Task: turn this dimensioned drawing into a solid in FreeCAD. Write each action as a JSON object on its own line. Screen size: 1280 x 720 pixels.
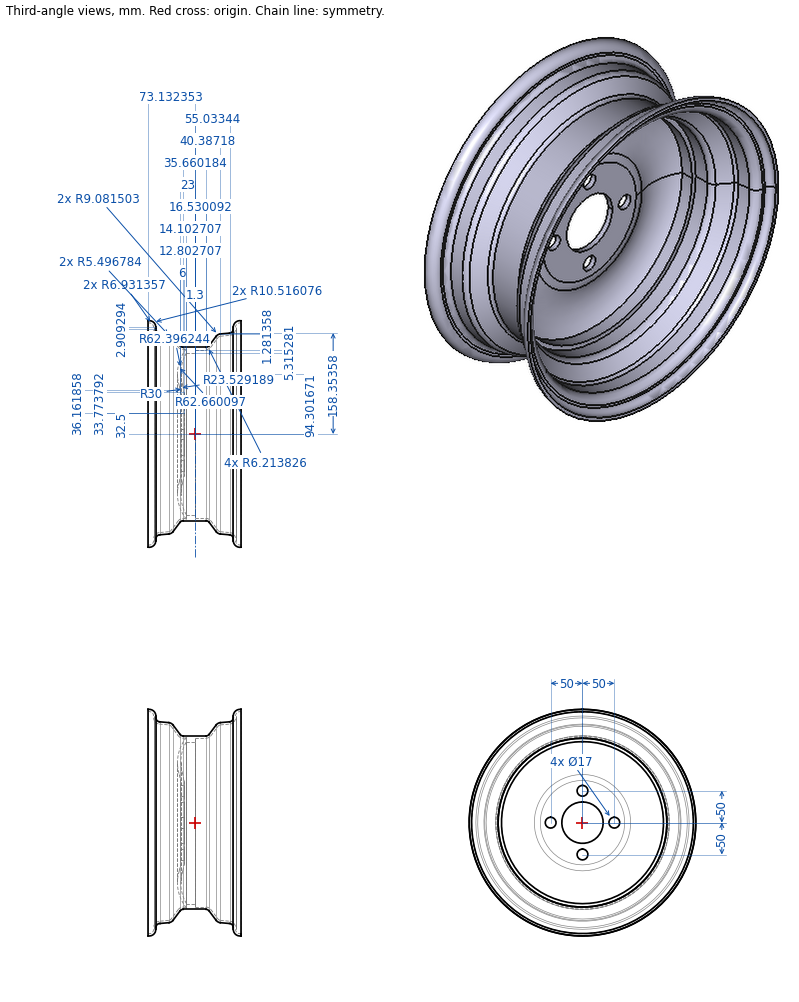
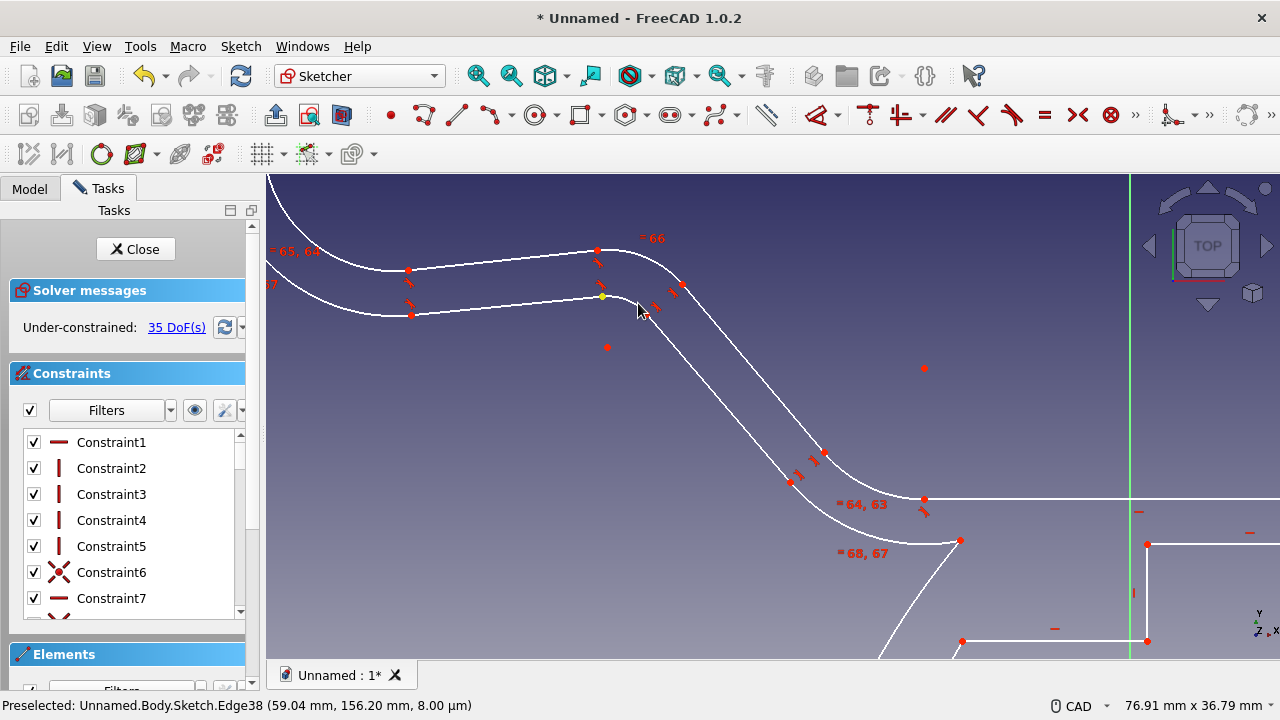
{"action": "left_click", "coordinate": [636, 305]}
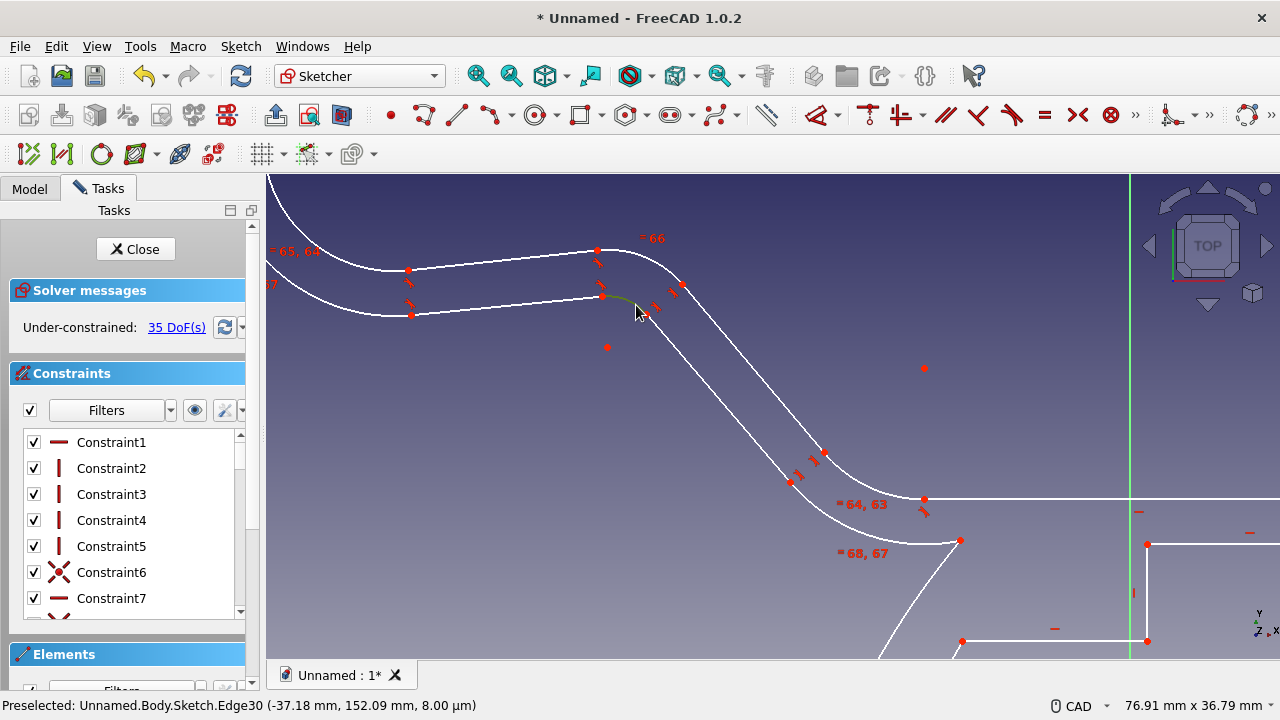
{"action": "scroll", "coordinate": [638, 303], "scroll_direction": "down", "scroll_amount": 10}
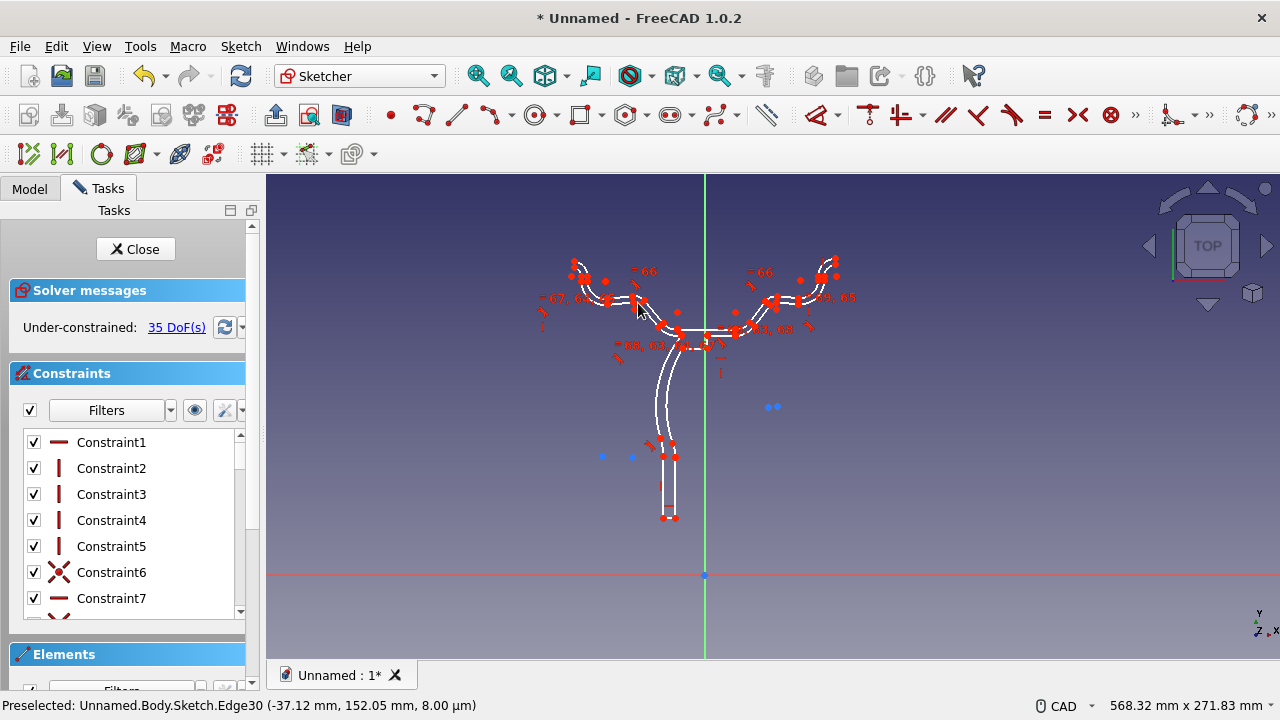
{"action": "scroll", "coordinate": [775, 303], "scroll_direction": "up", "scroll_amount": 10}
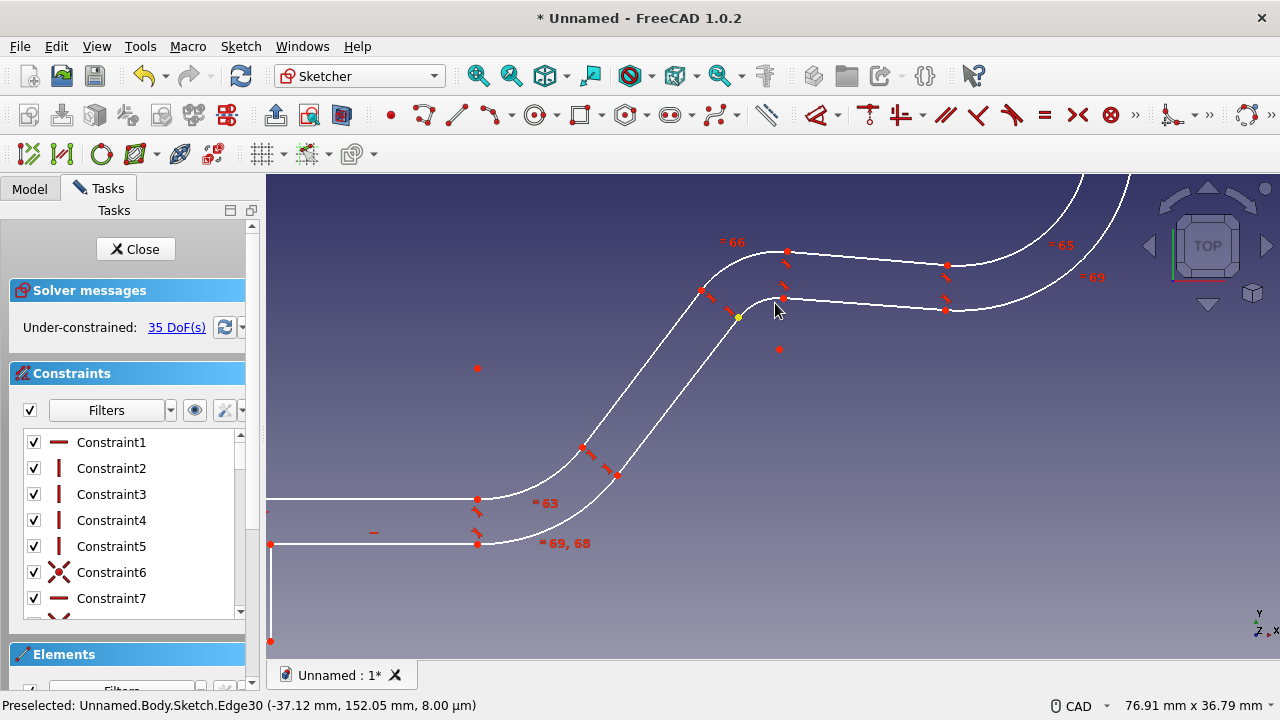
{"action": "left_click", "coordinate": [768, 299]}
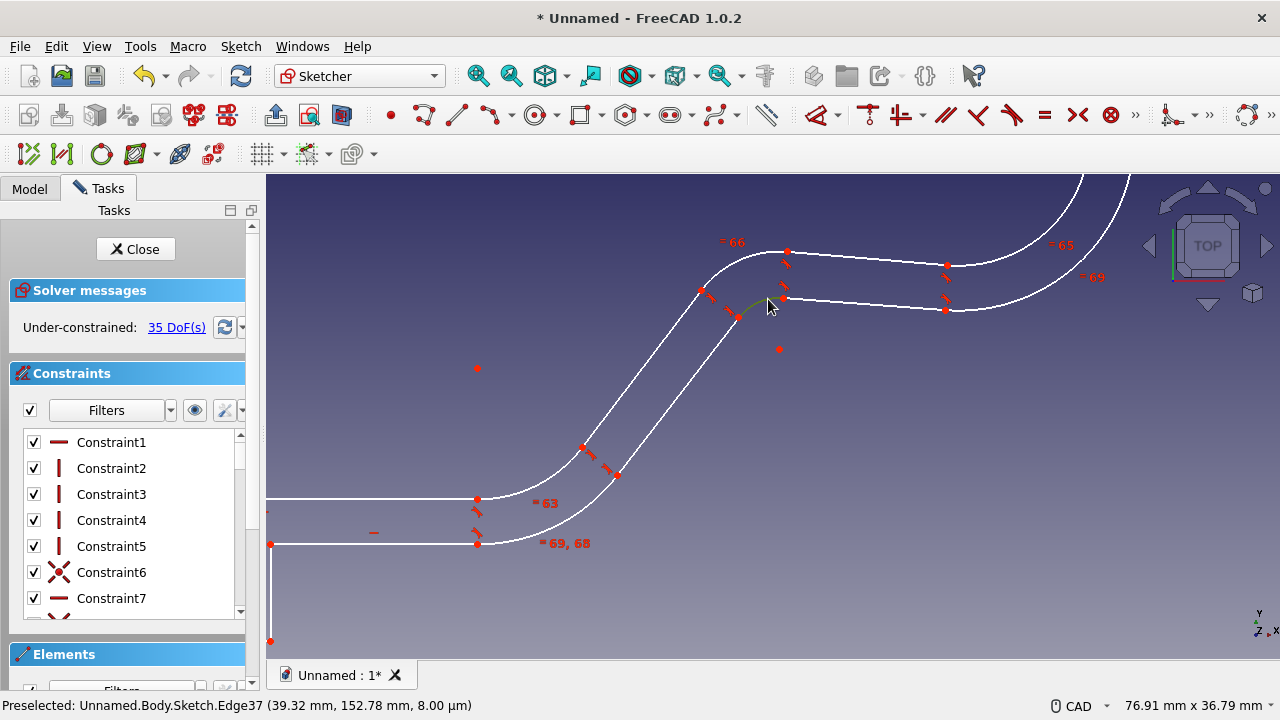
{"action": "key", "text": "e"}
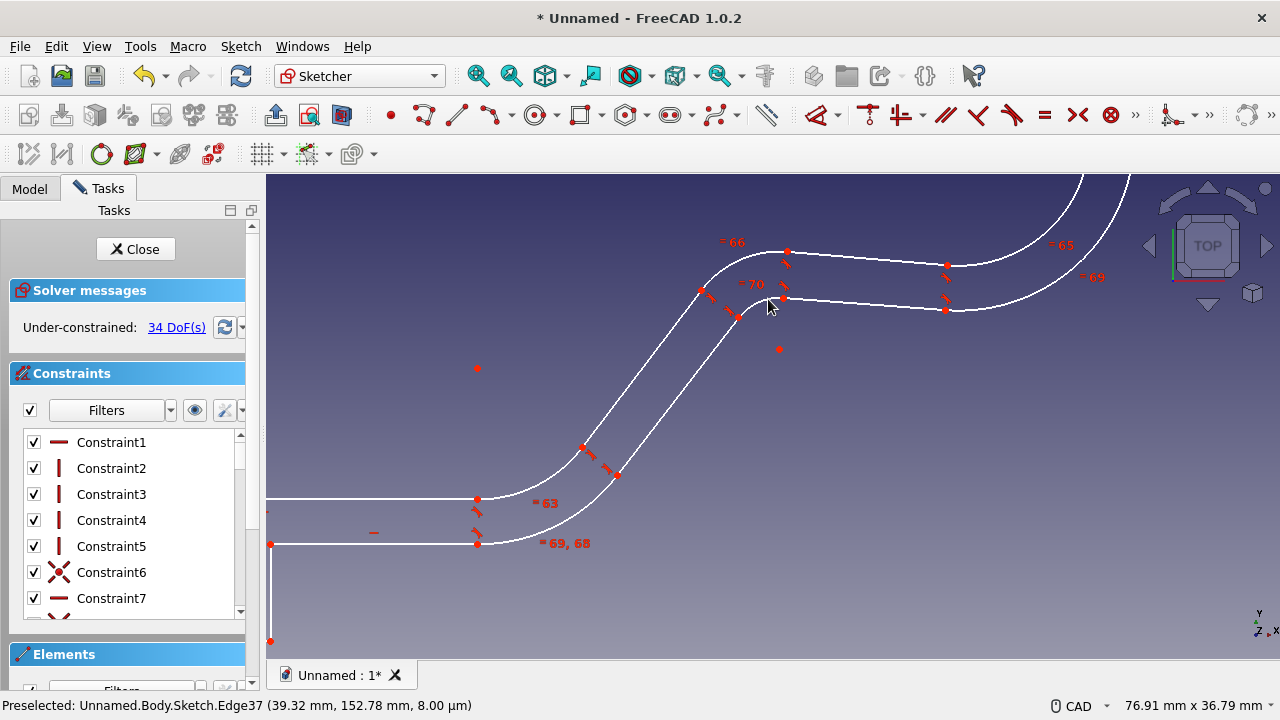
{"action": "scroll", "coordinate": [775, 303], "scroll_direction": "down", "scroll_amount": 10}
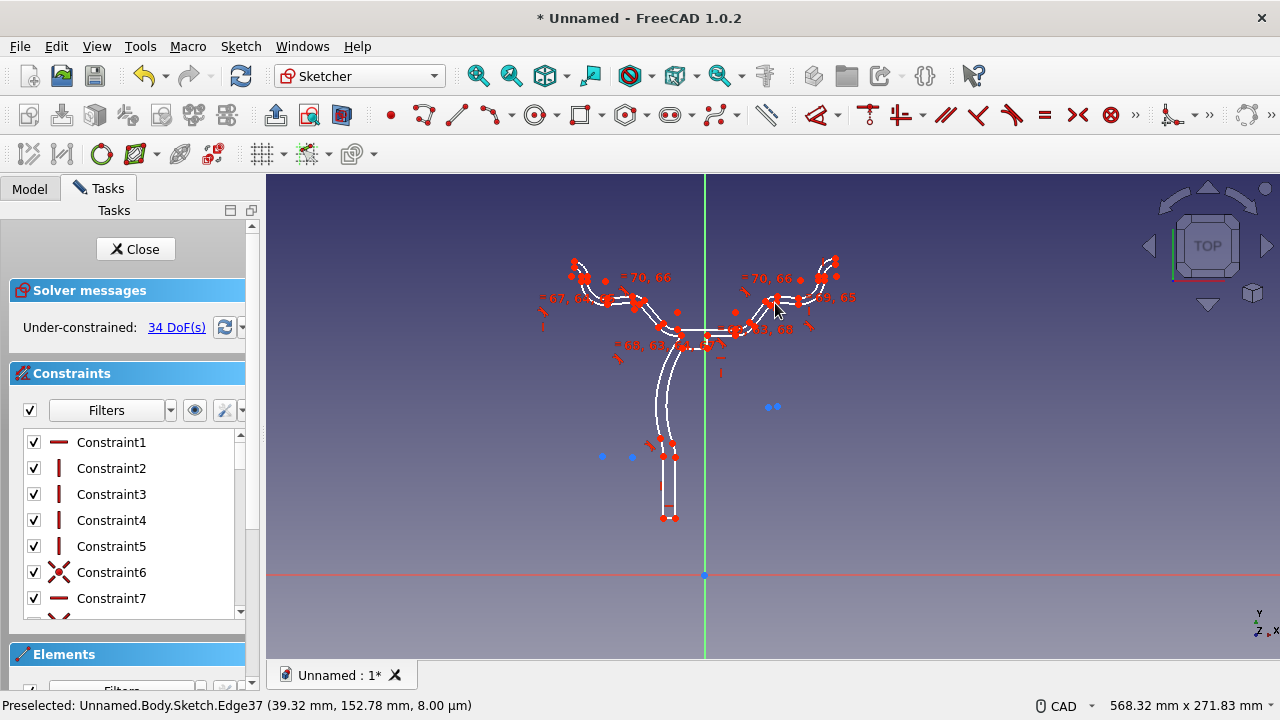
{"action": "scroll", "coordinate": [581, 273], "scroll_direction": "up", "scroll_amount": 7}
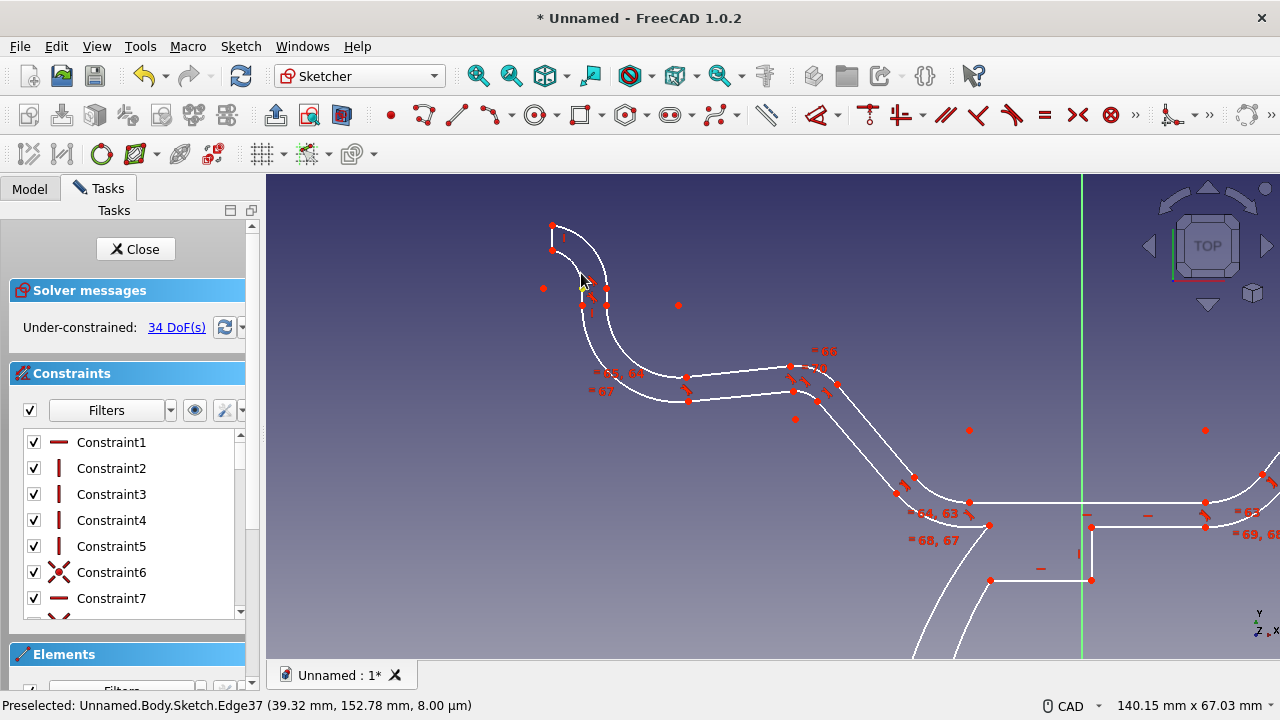
{"action": "left_click", "coordinate": [579, 273]}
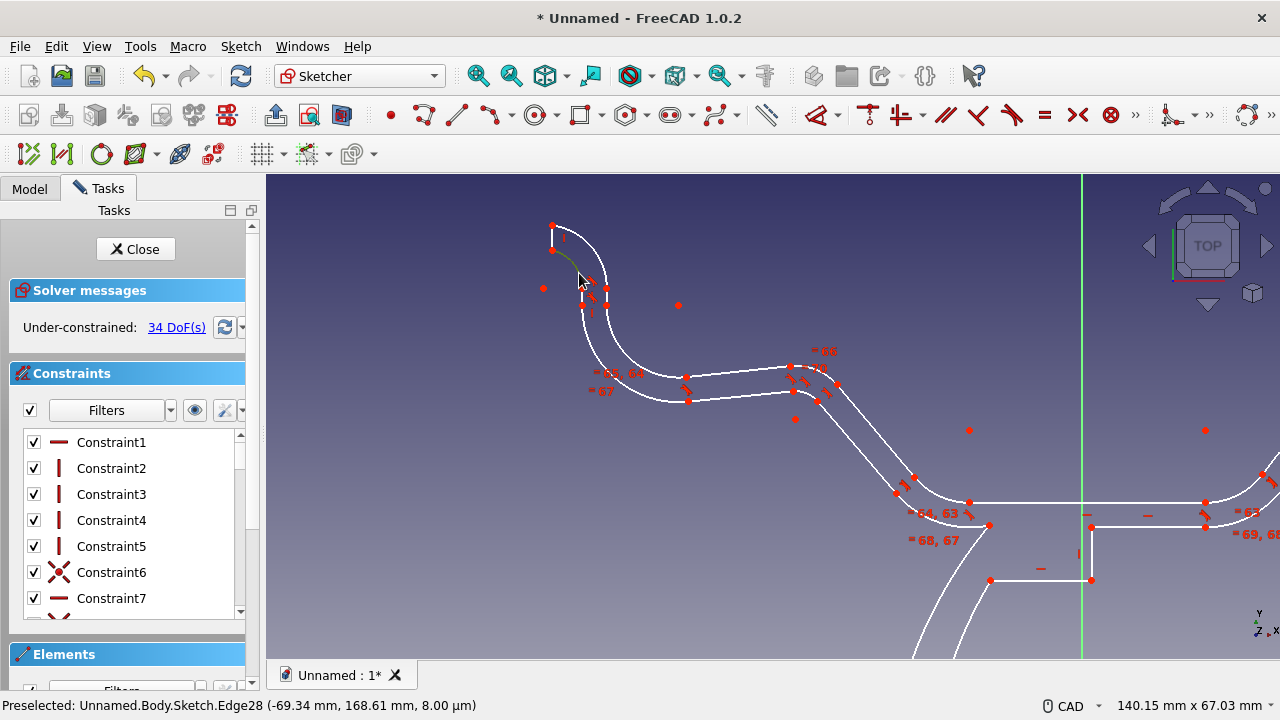
{"action": "scroll", "coordinate": [581, 273], "scroll_direction": "down", "scroll_amount": 7}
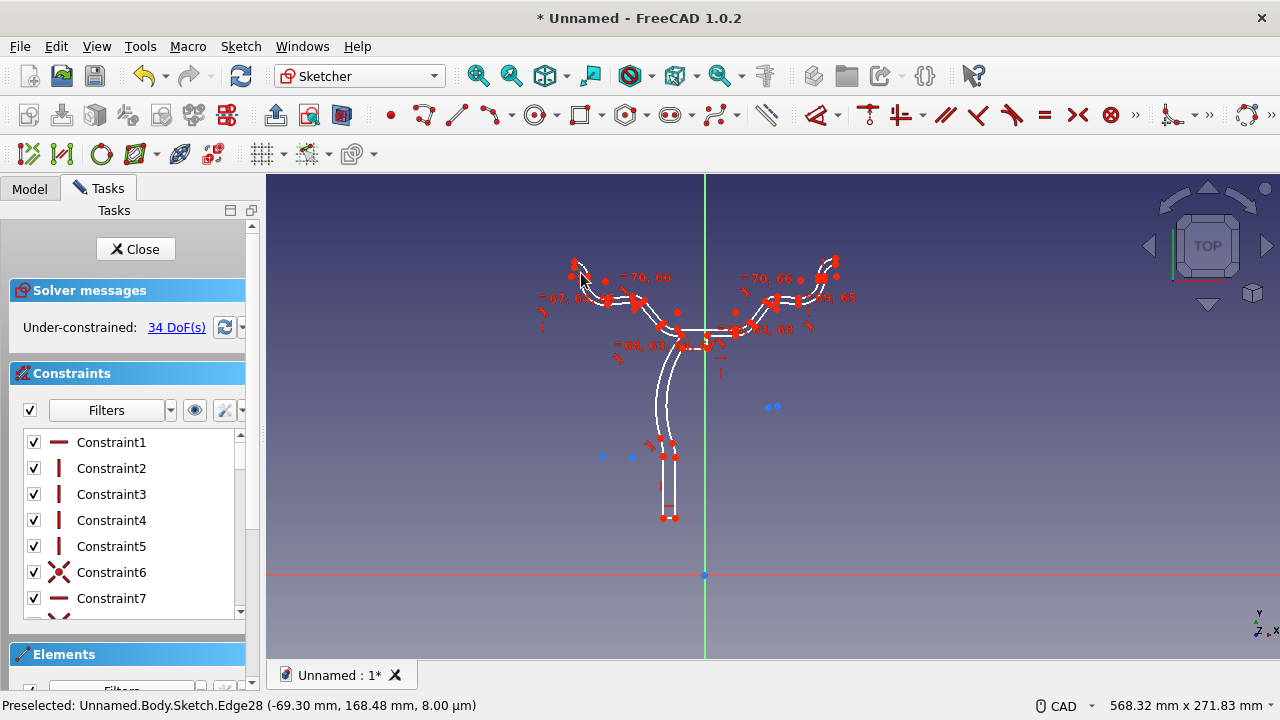
{"action": "scroll", "coordinate": [830, 266], "scroll_direction": "up", "scroll_amount": 5}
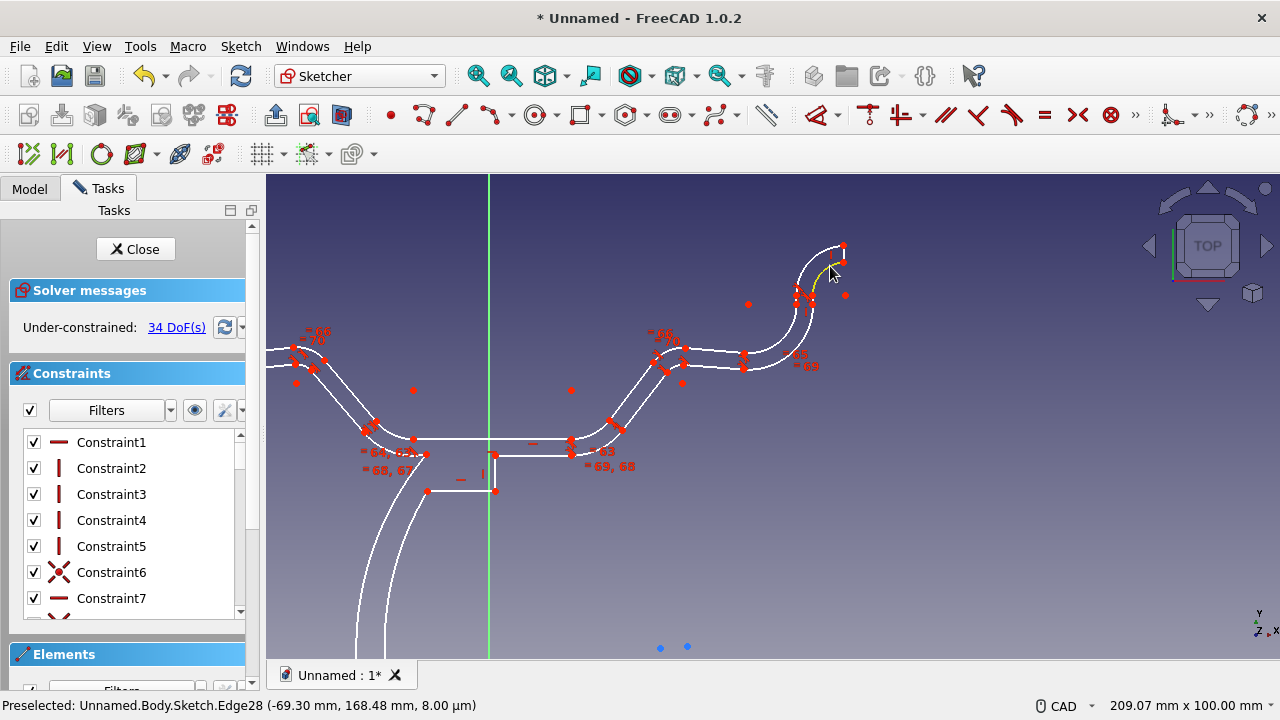
{"action": "left_click", "coordinate": [830, 267]}